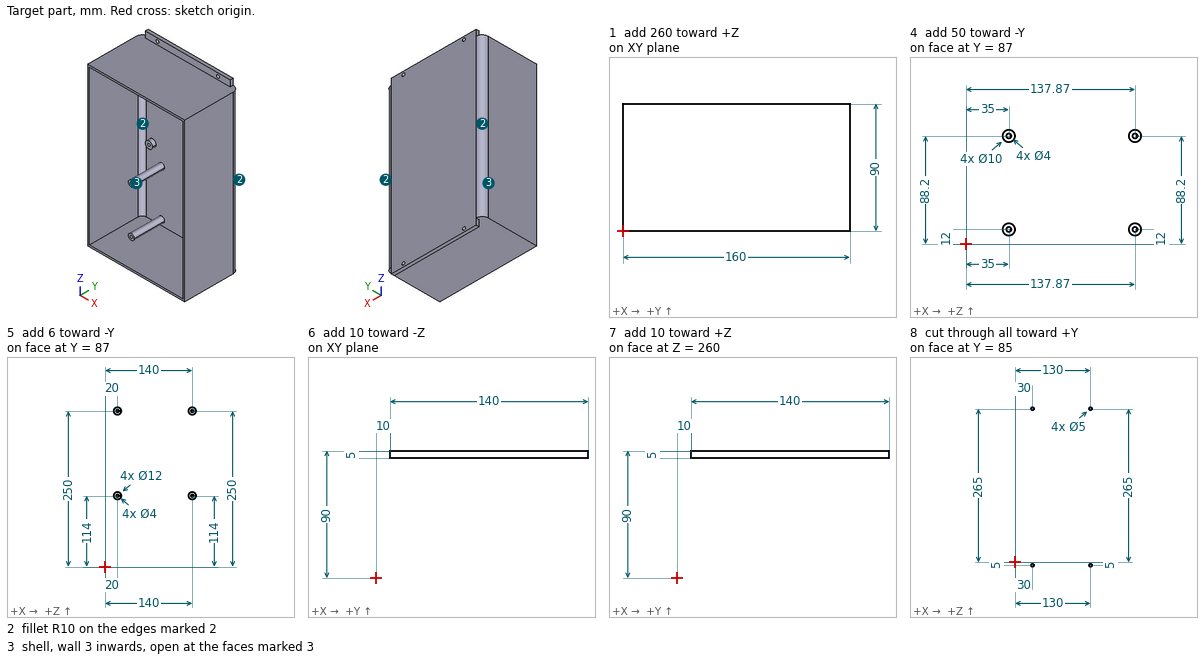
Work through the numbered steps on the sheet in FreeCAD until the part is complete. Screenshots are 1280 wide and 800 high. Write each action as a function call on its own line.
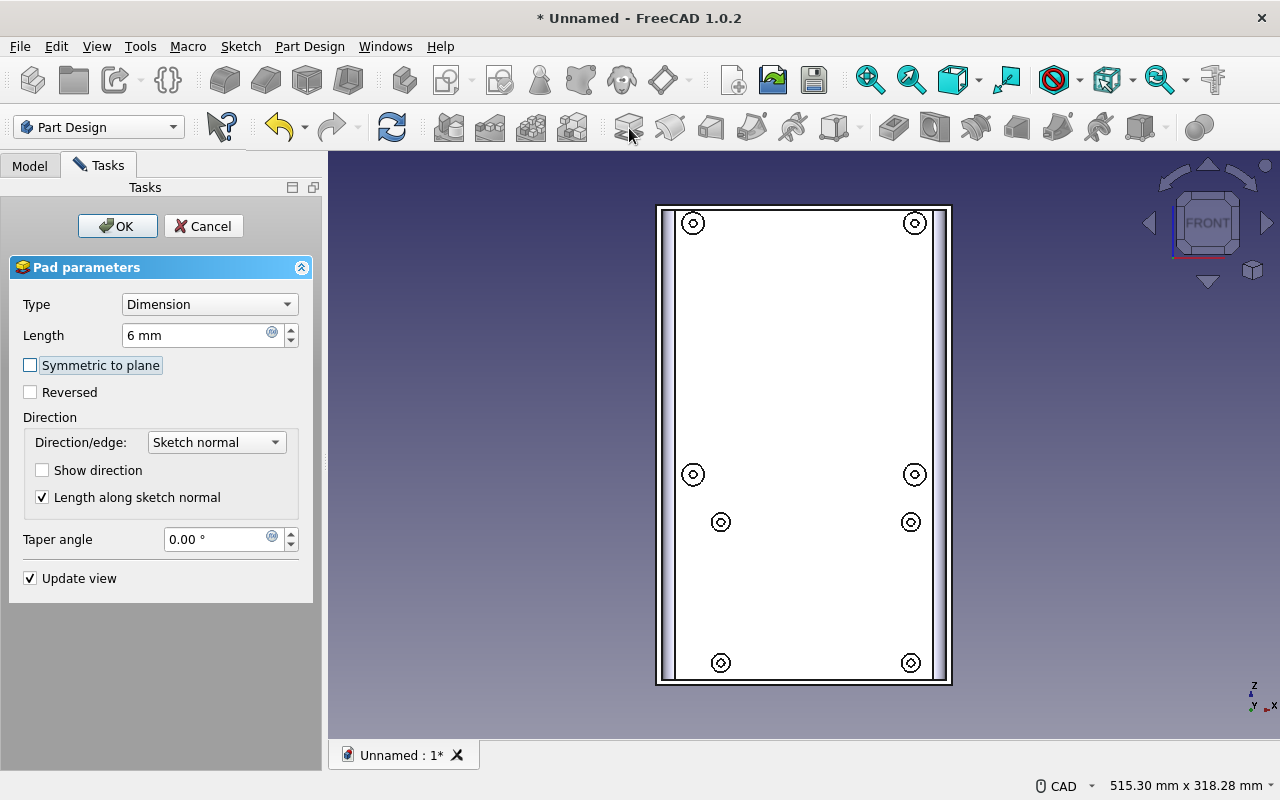
click(118, 226)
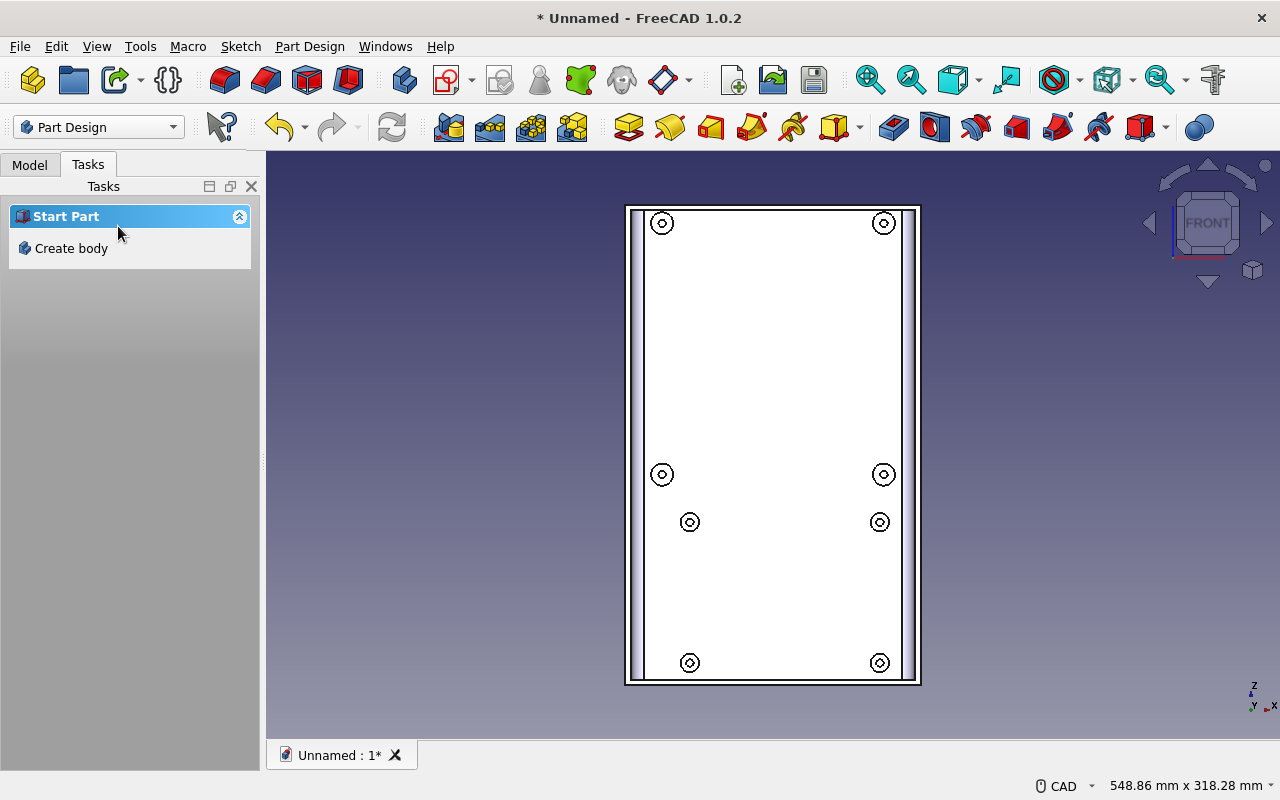
click(446, 80)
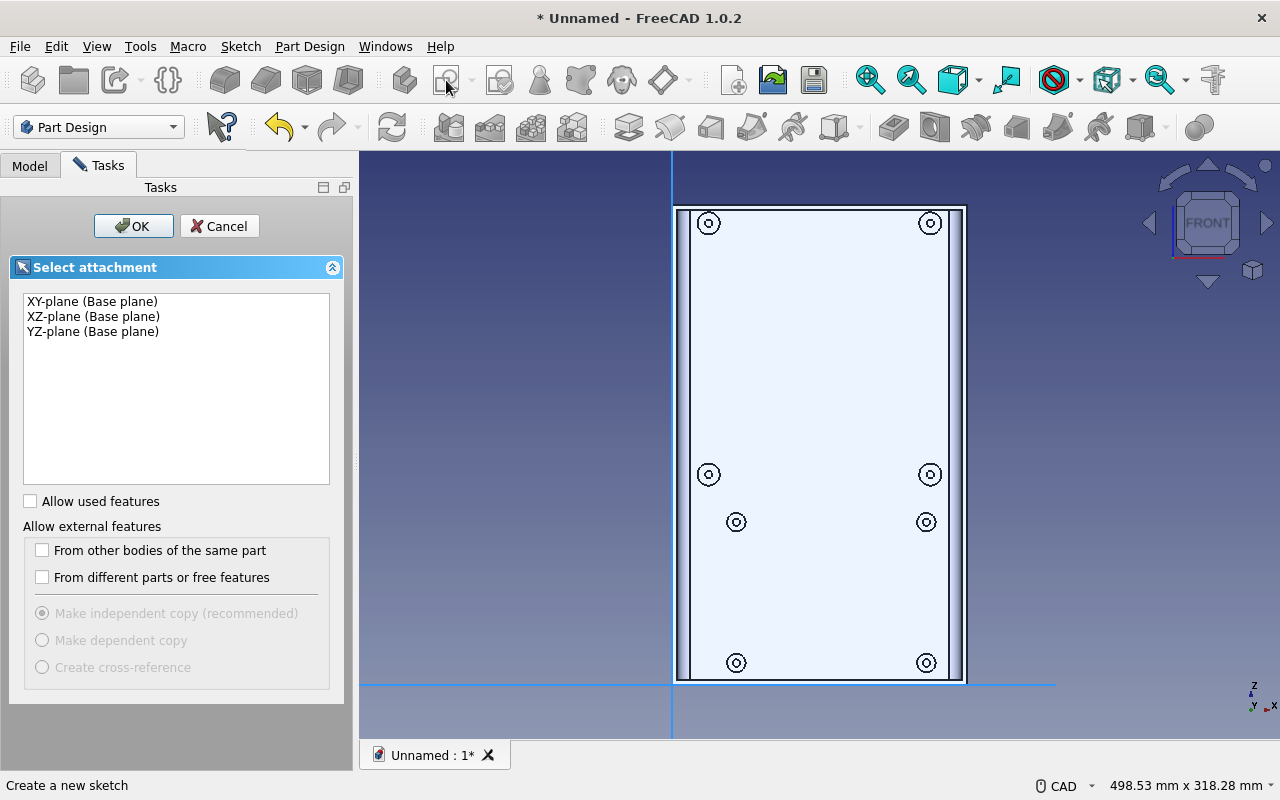
click(84, 302)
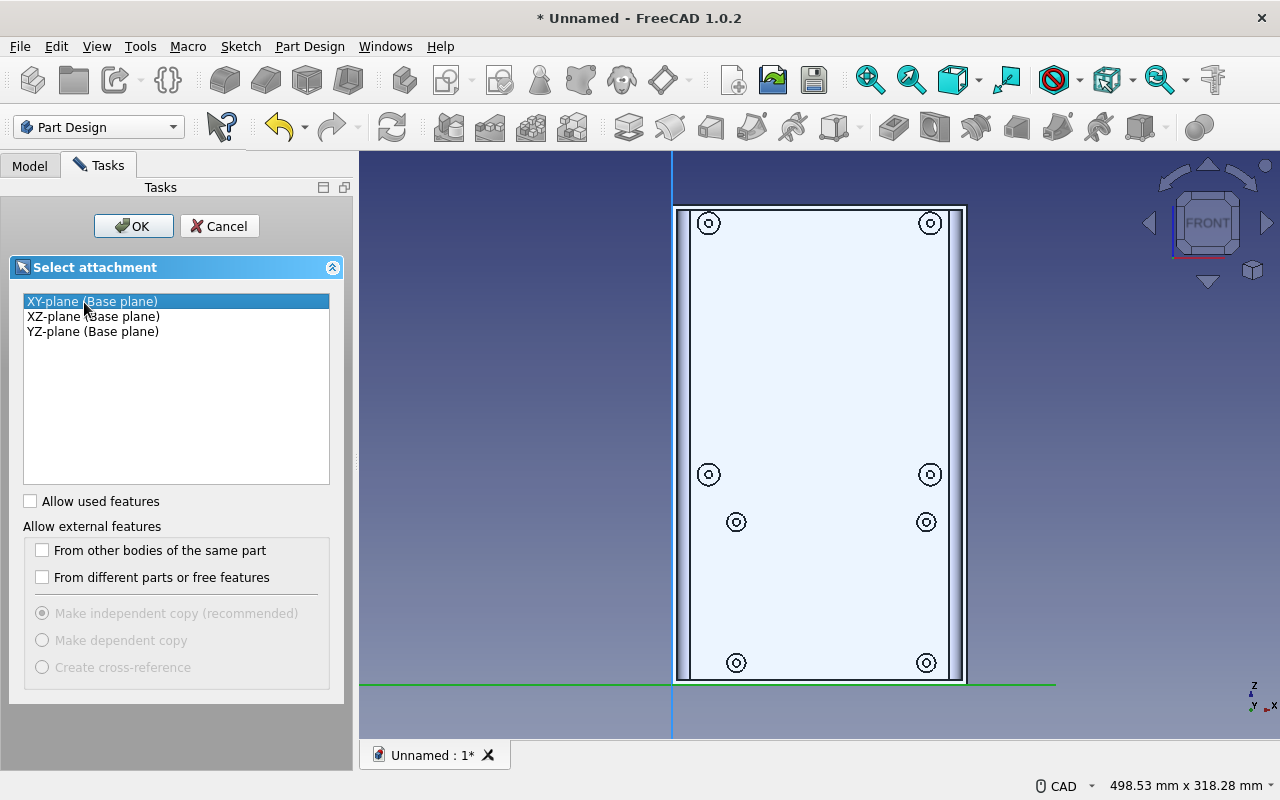
click(134, 226)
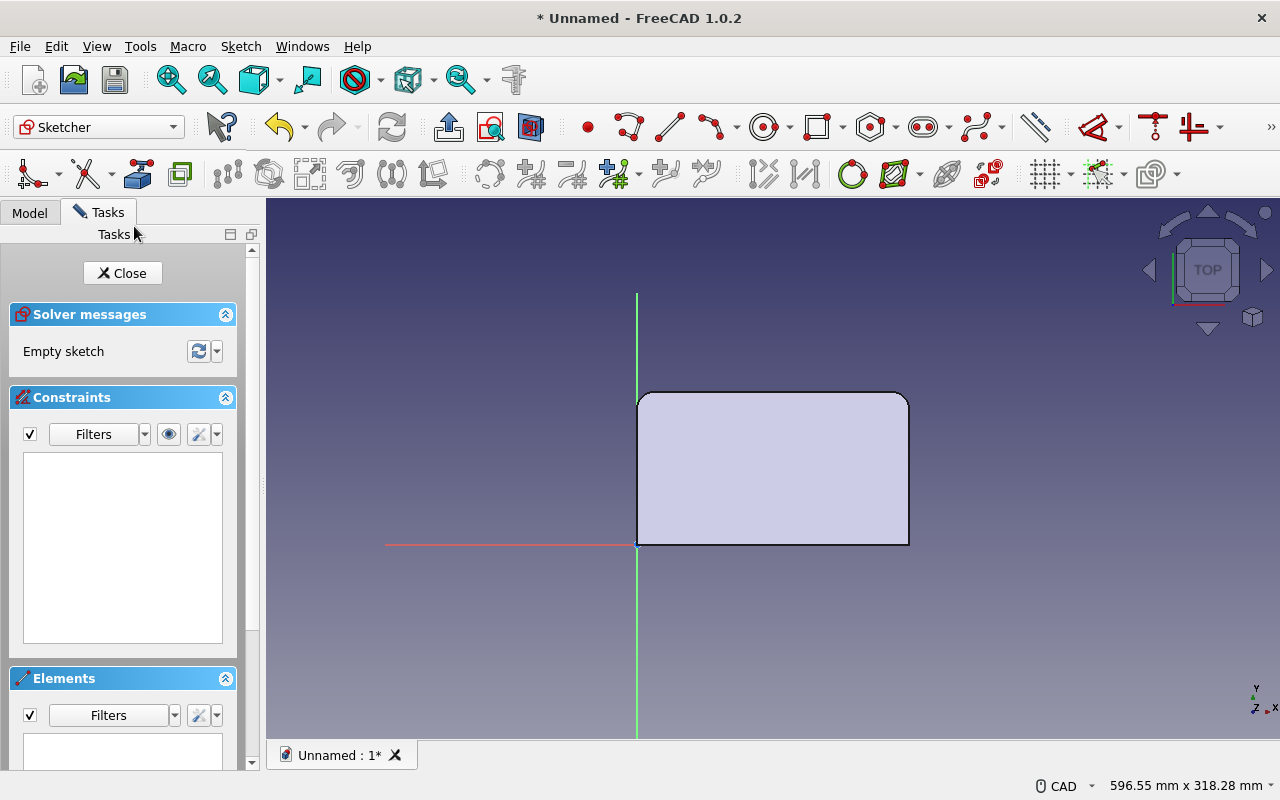
click(531, 128)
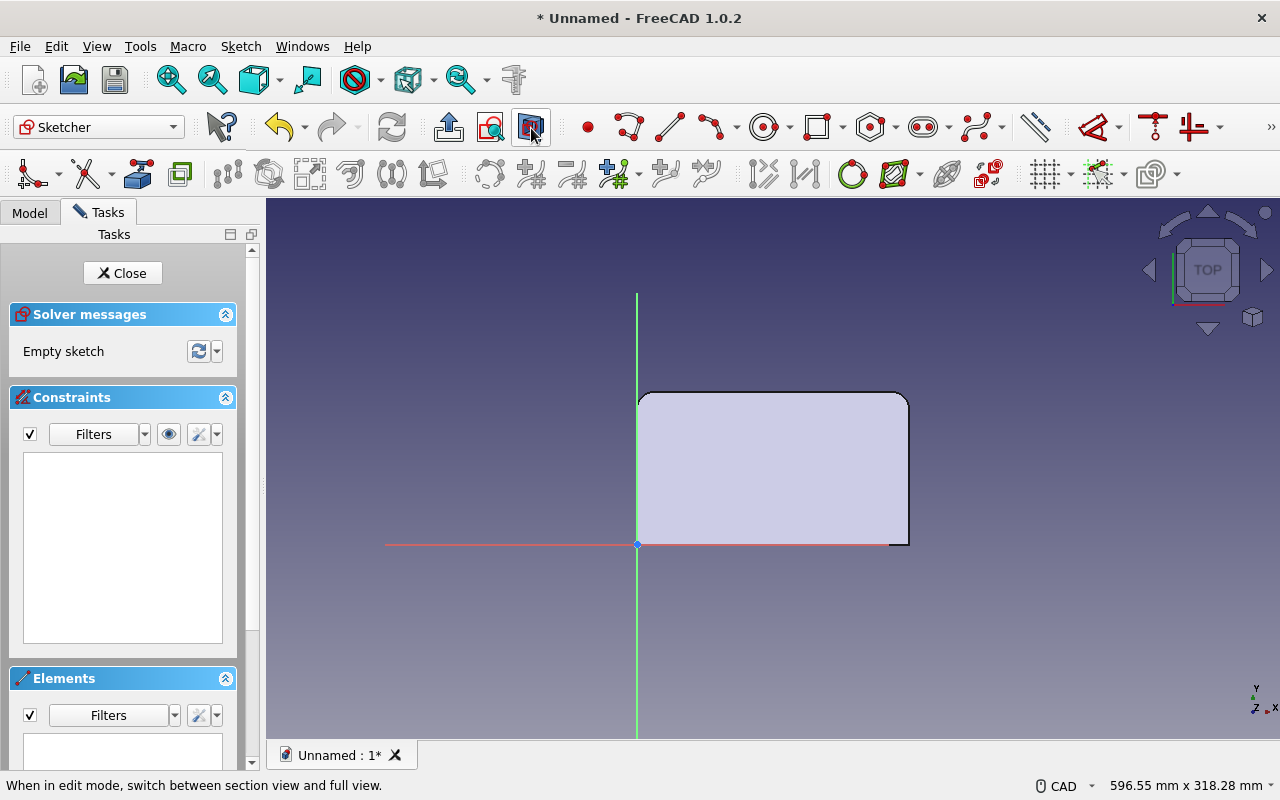
scroll(813, 468, up, 4)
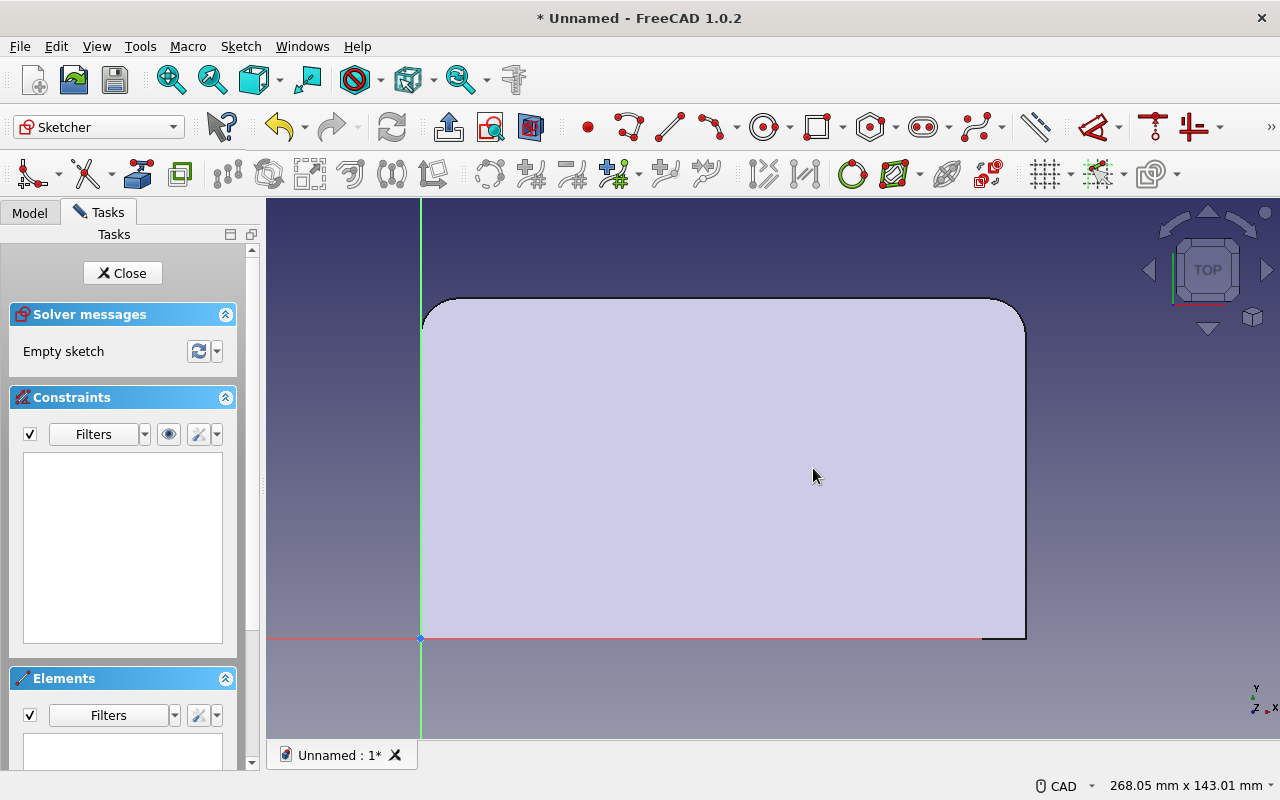
click(816, 128)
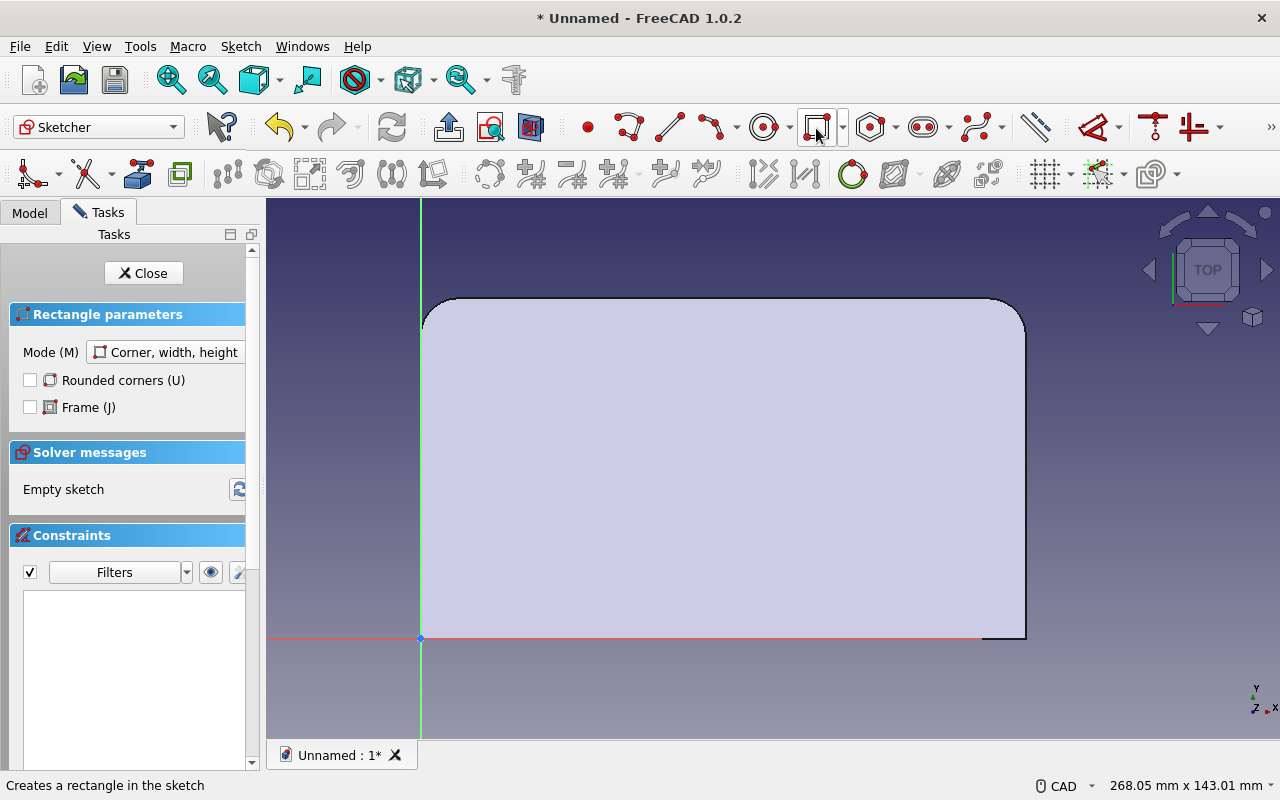
click(459, 298)
click(988, 317)
key(Escape)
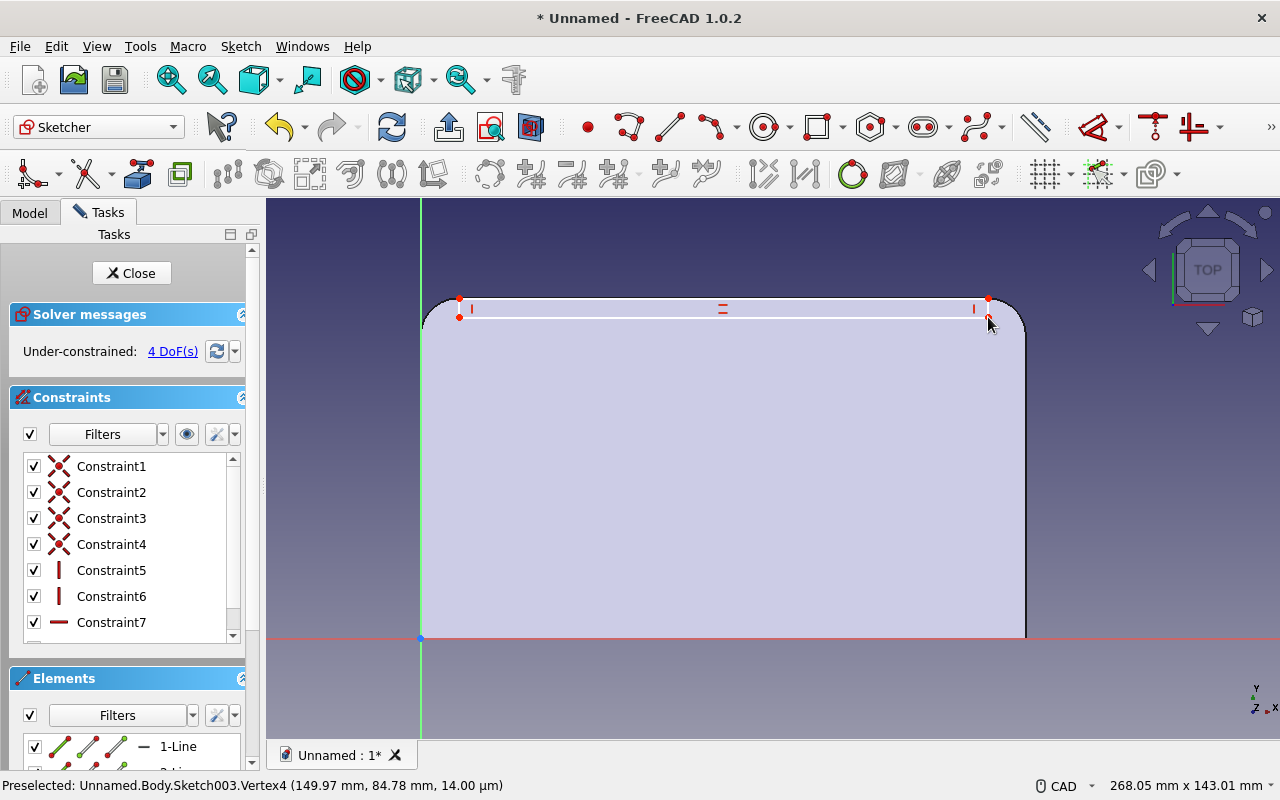
click(1092, 128)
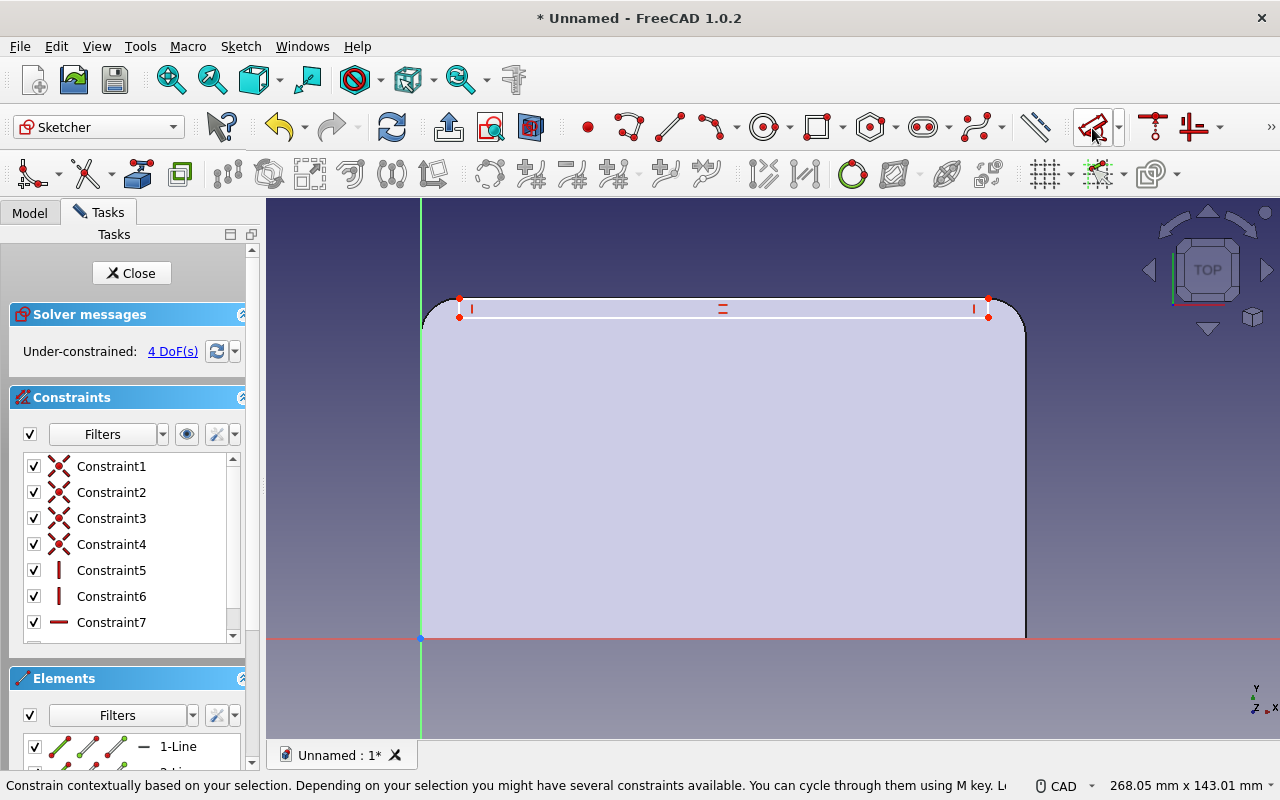
scroll(459, 308, up, 4)